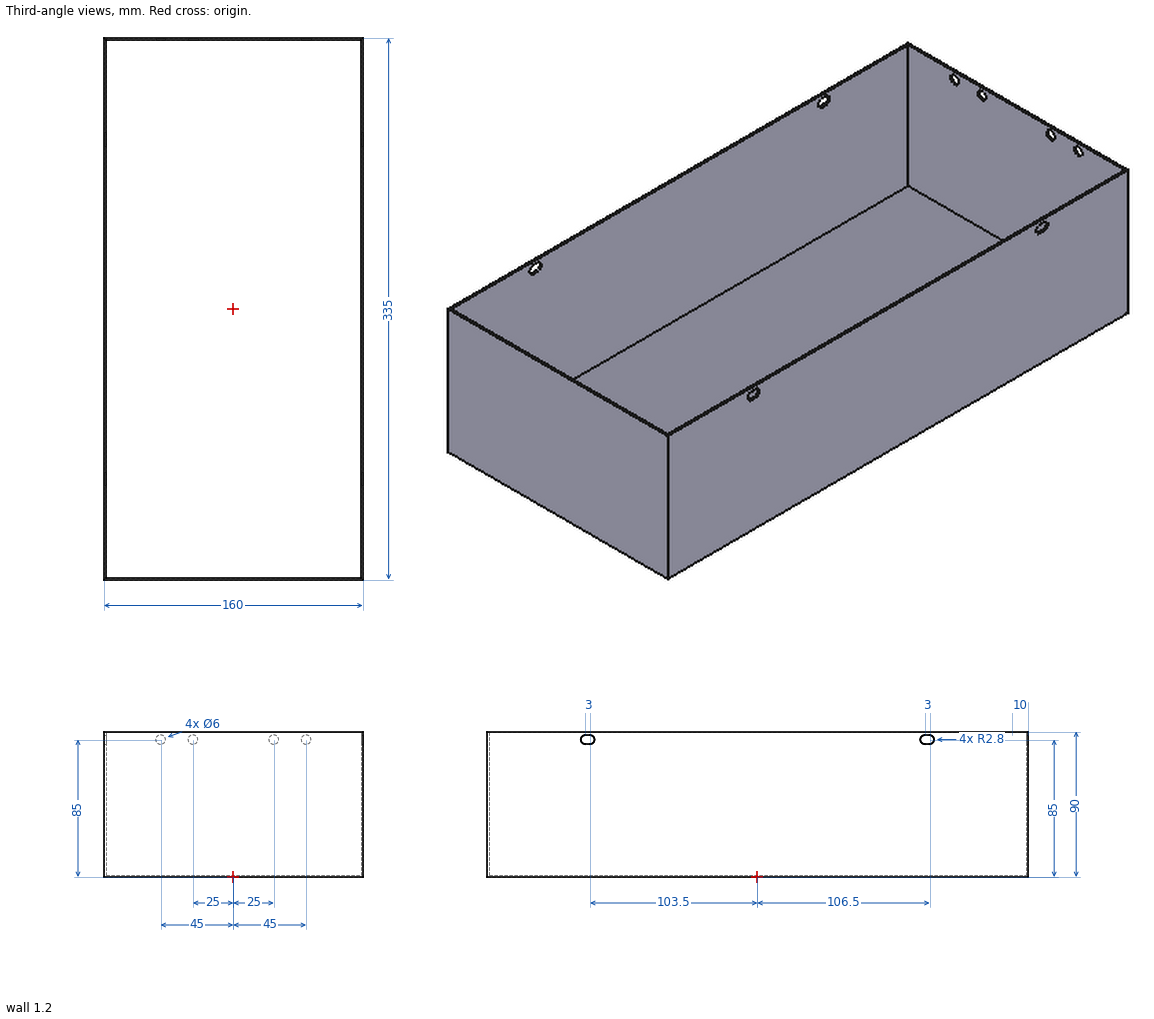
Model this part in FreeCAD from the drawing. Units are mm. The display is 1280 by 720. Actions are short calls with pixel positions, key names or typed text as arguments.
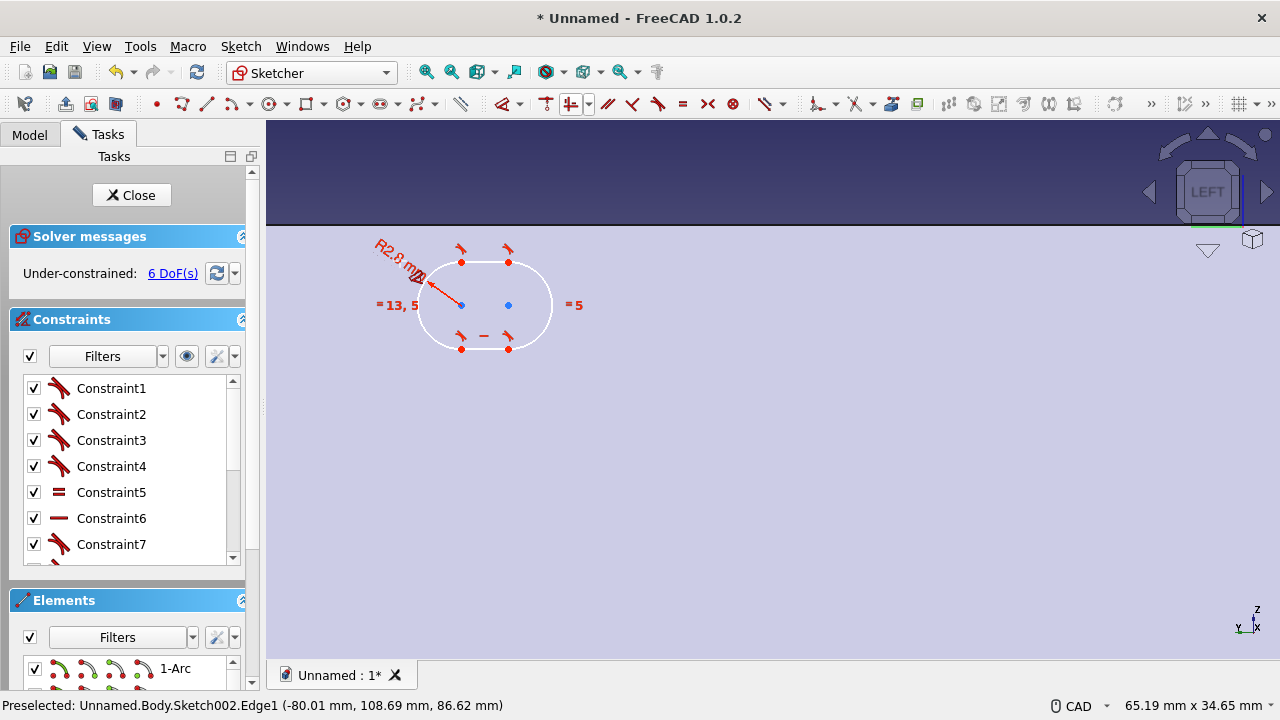
click(475, 262)
click(485, 228)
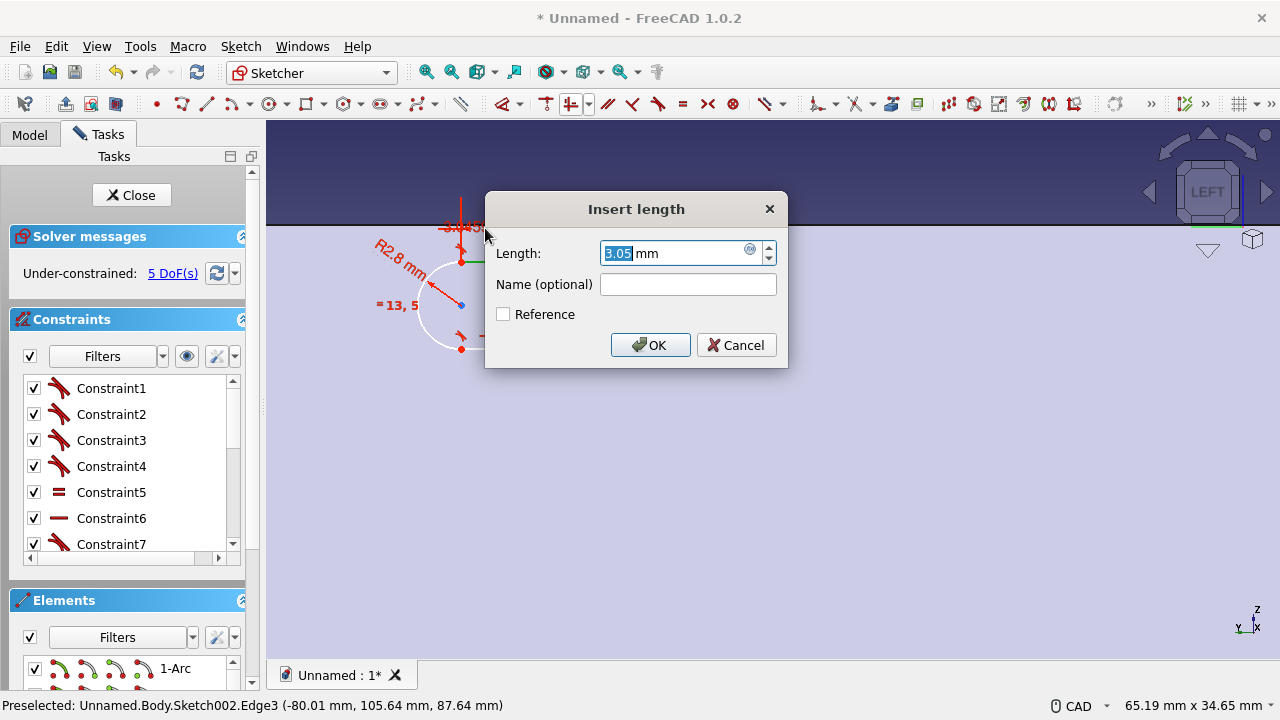
text(3)
key(Return)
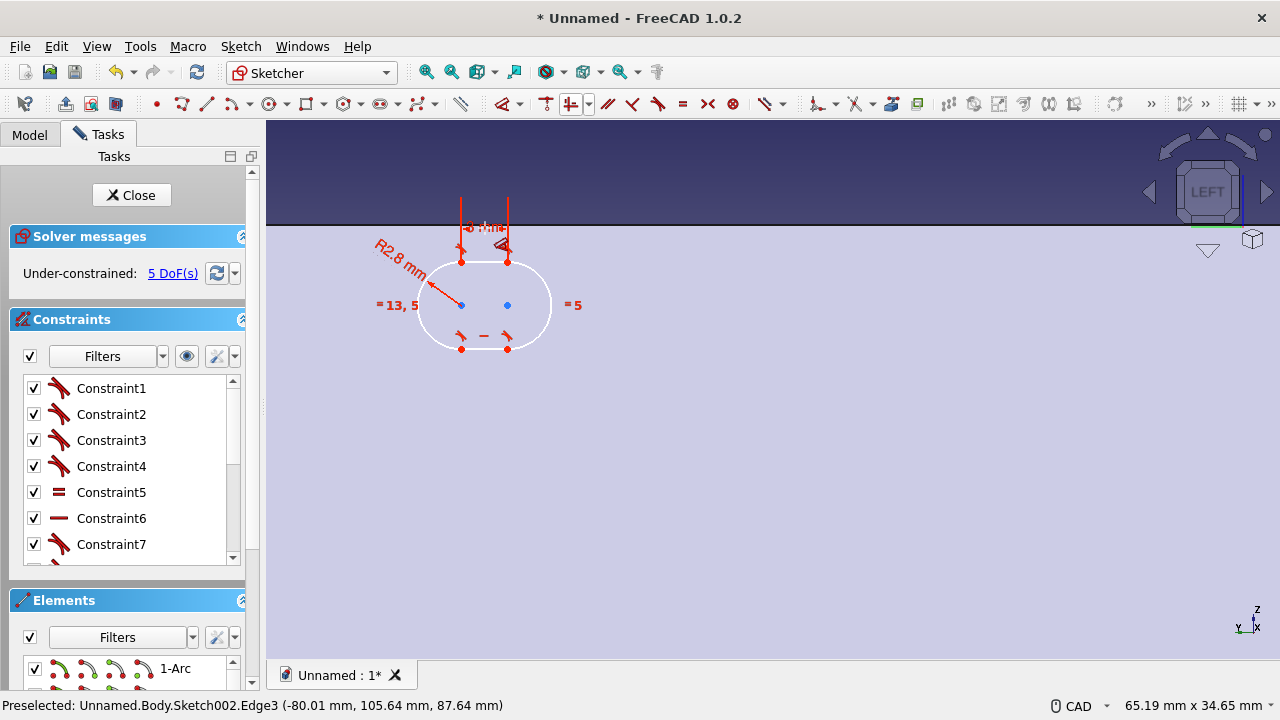
scroll(425, 280, down, 9)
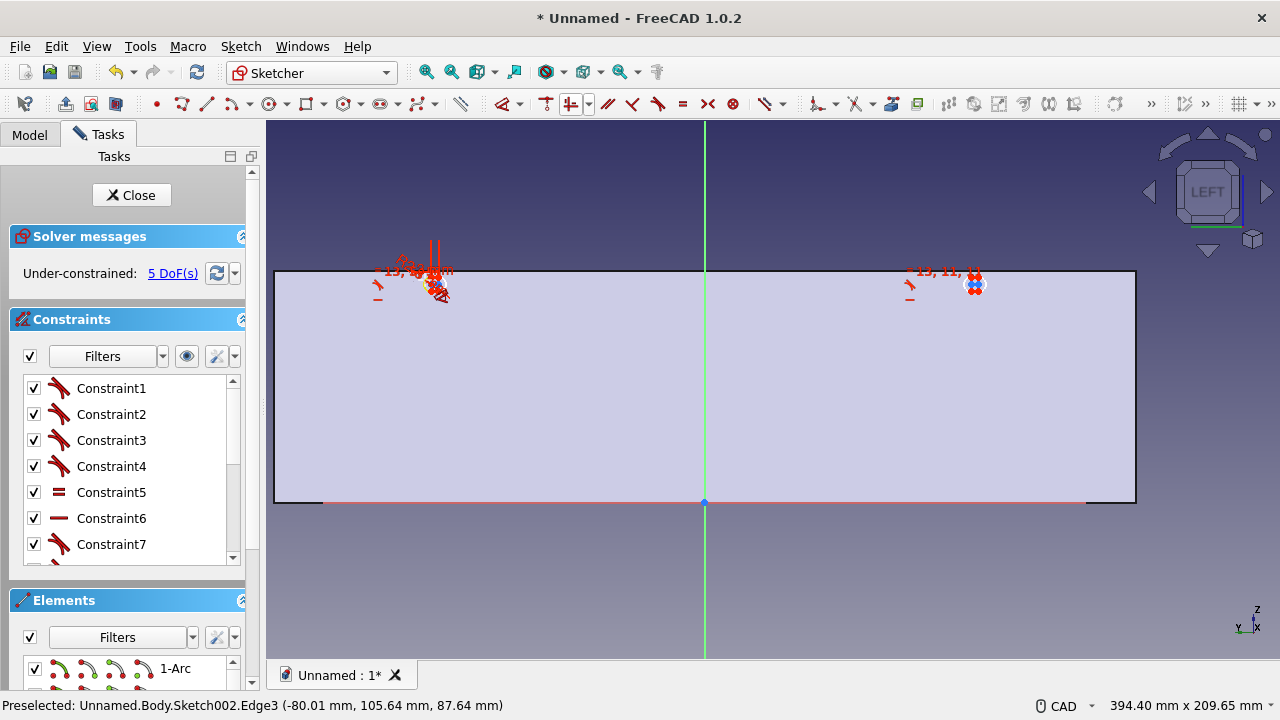
scroll(973, 277, up, 10)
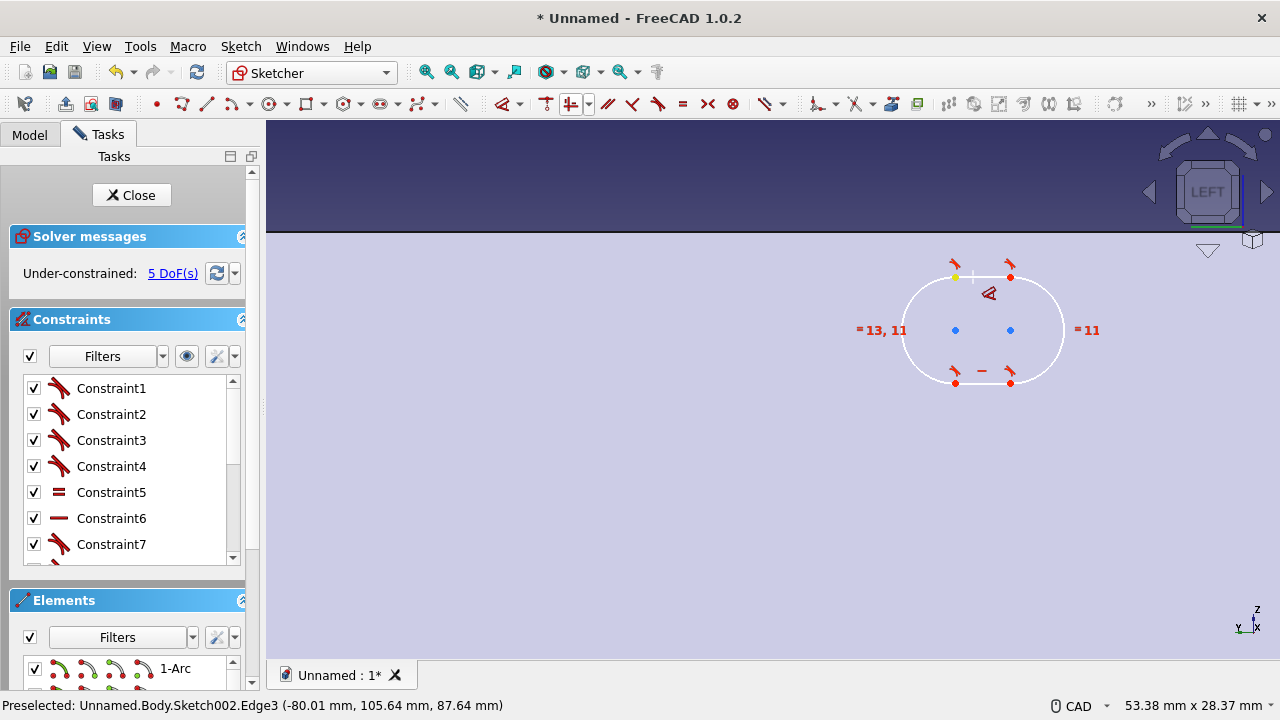
click(972, 277)
click(983, 243)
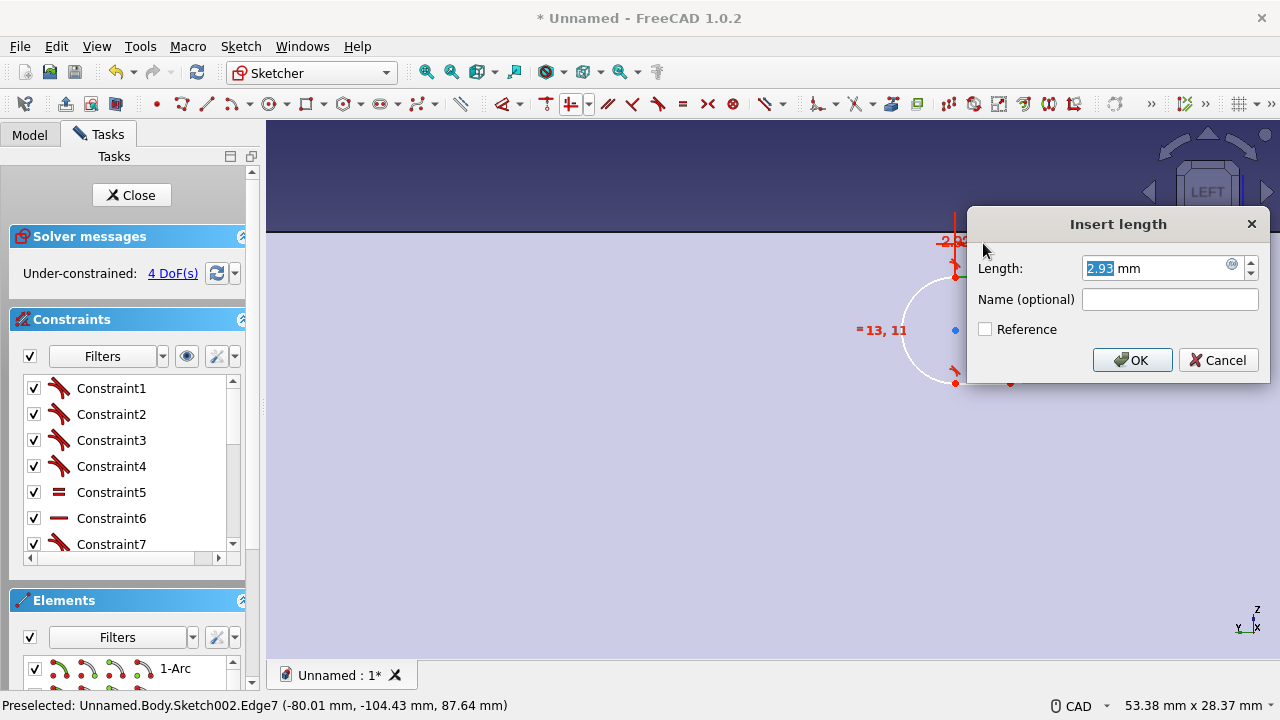
text(3)
key(Return)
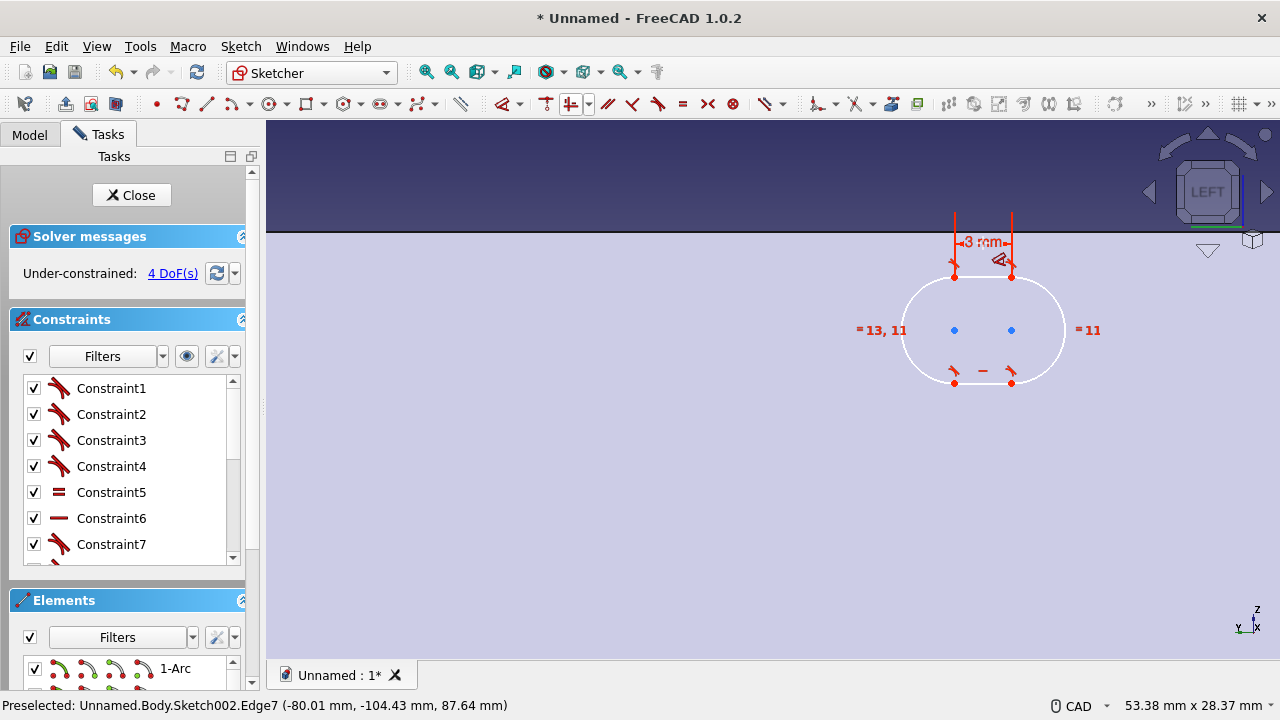
scroll(973, 277, down, 10)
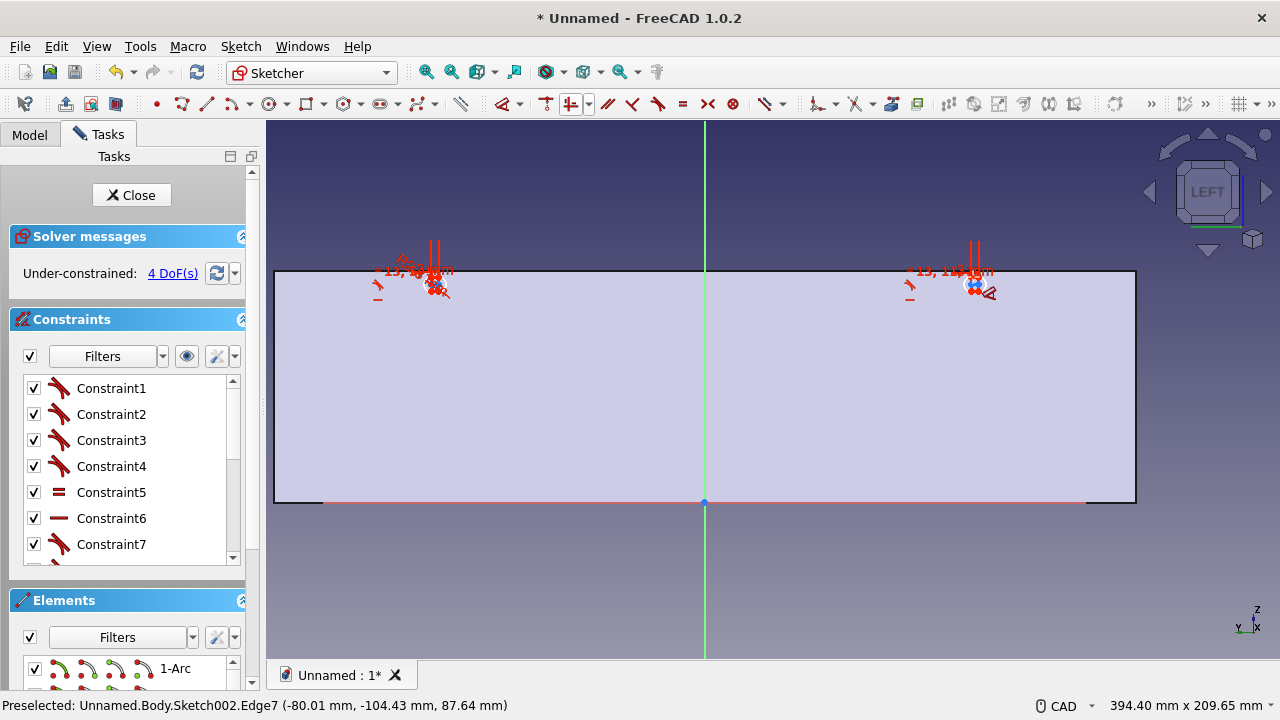
scroll(431, 284, up, 3)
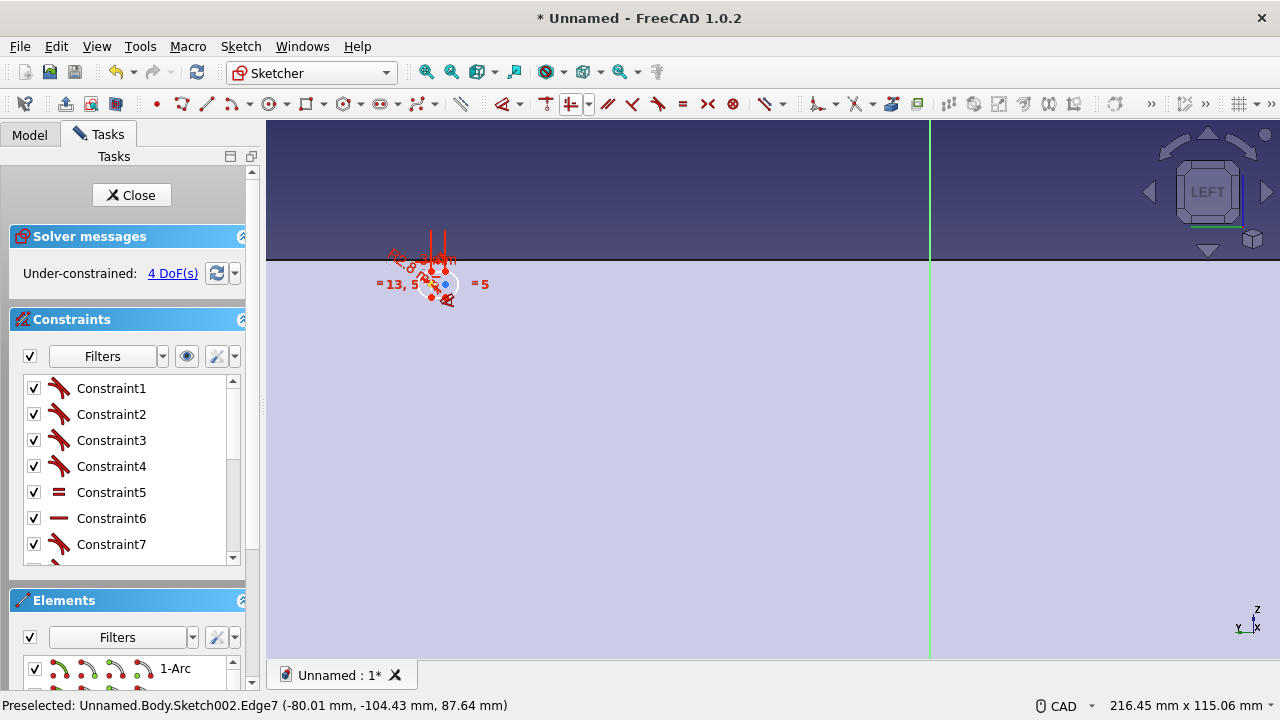
click(431, 285)
click(397, 458)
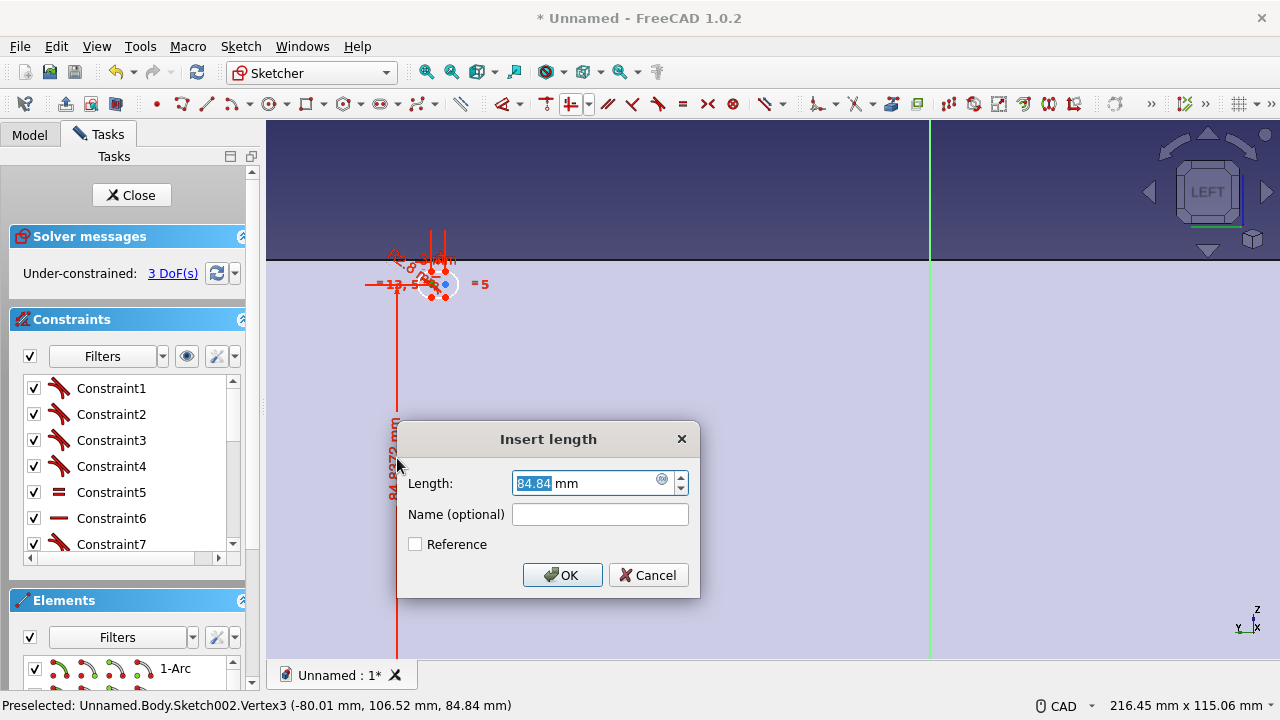
text(85)
key(Return)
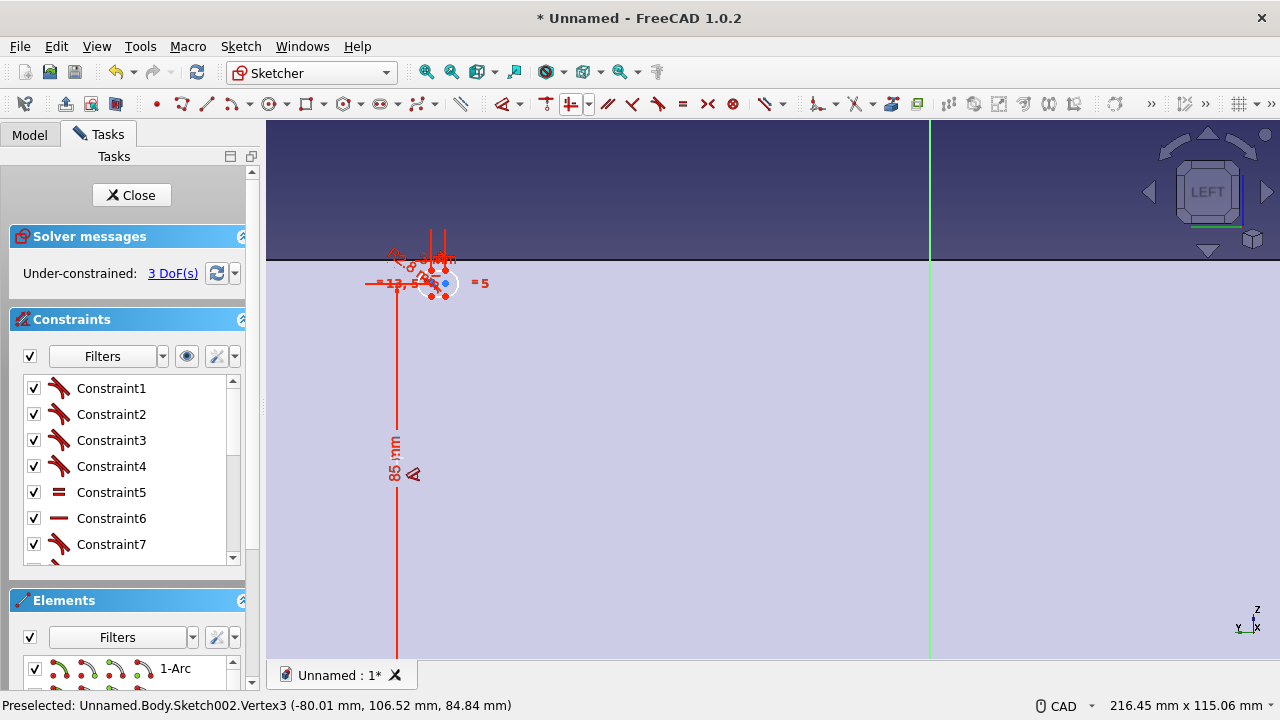
scroll(430, 284, down, 3)